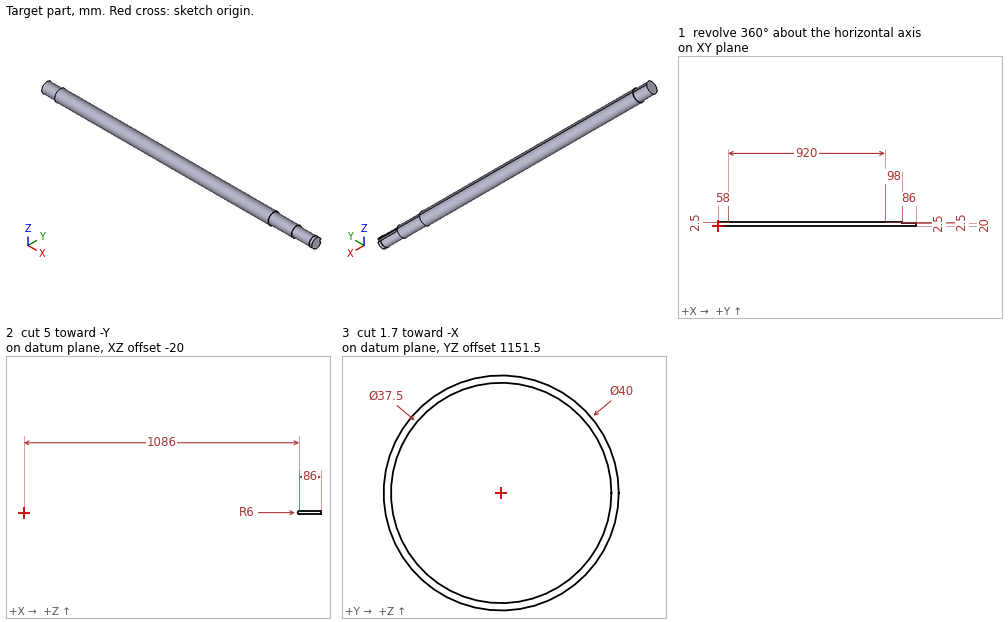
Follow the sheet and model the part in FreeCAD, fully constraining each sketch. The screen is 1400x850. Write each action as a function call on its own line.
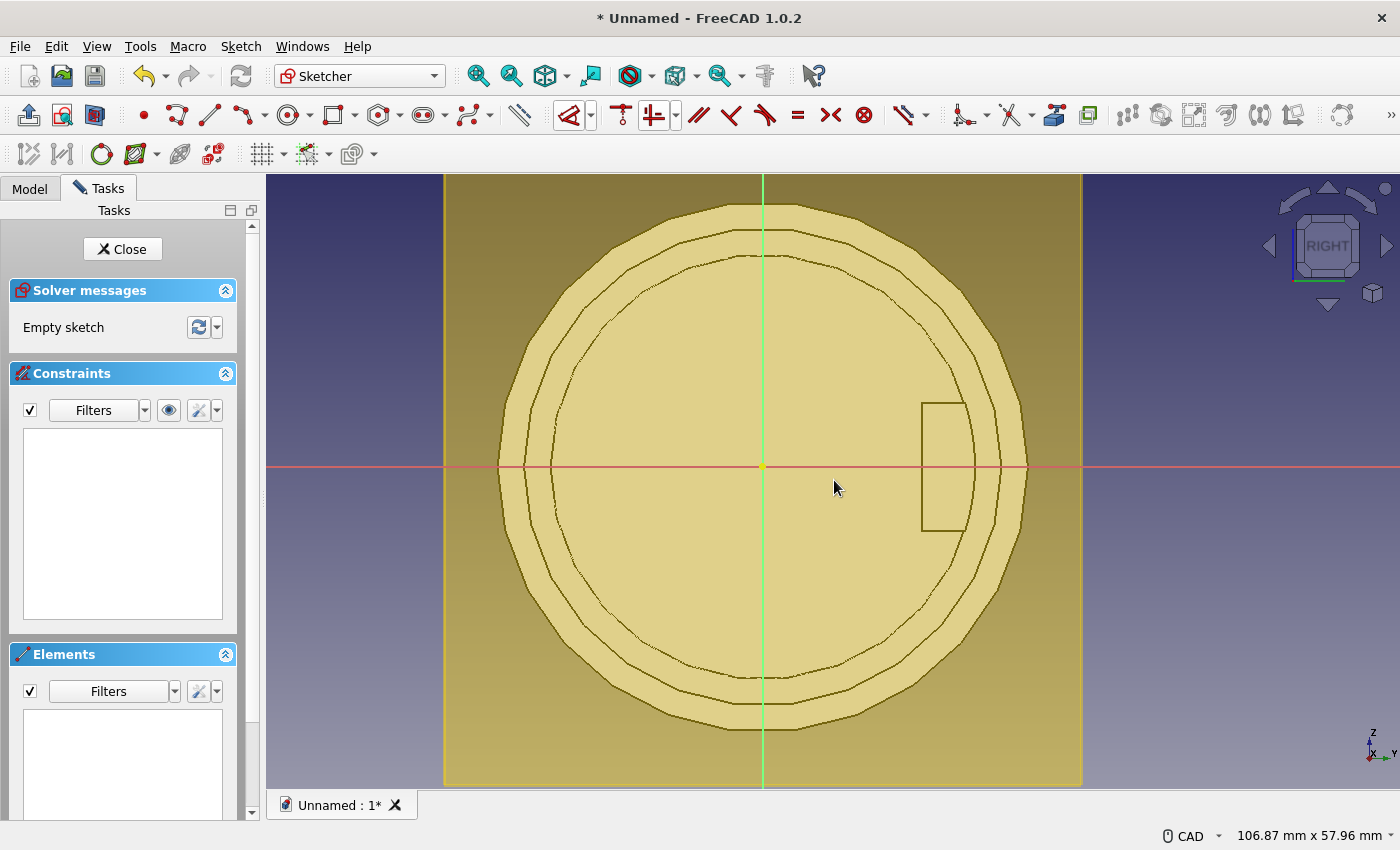
click(288, 116)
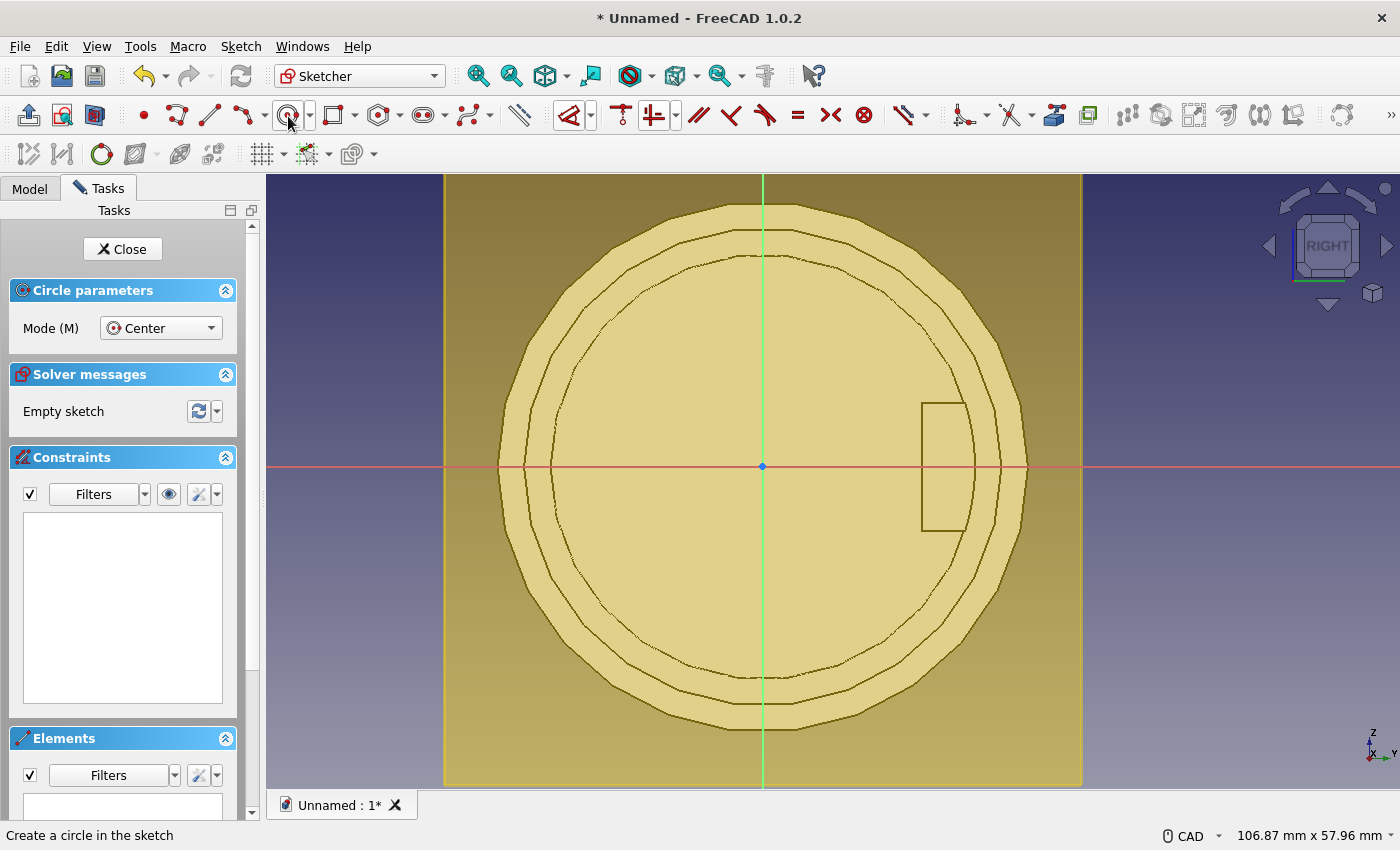
click(763, 467)
click(913, 317)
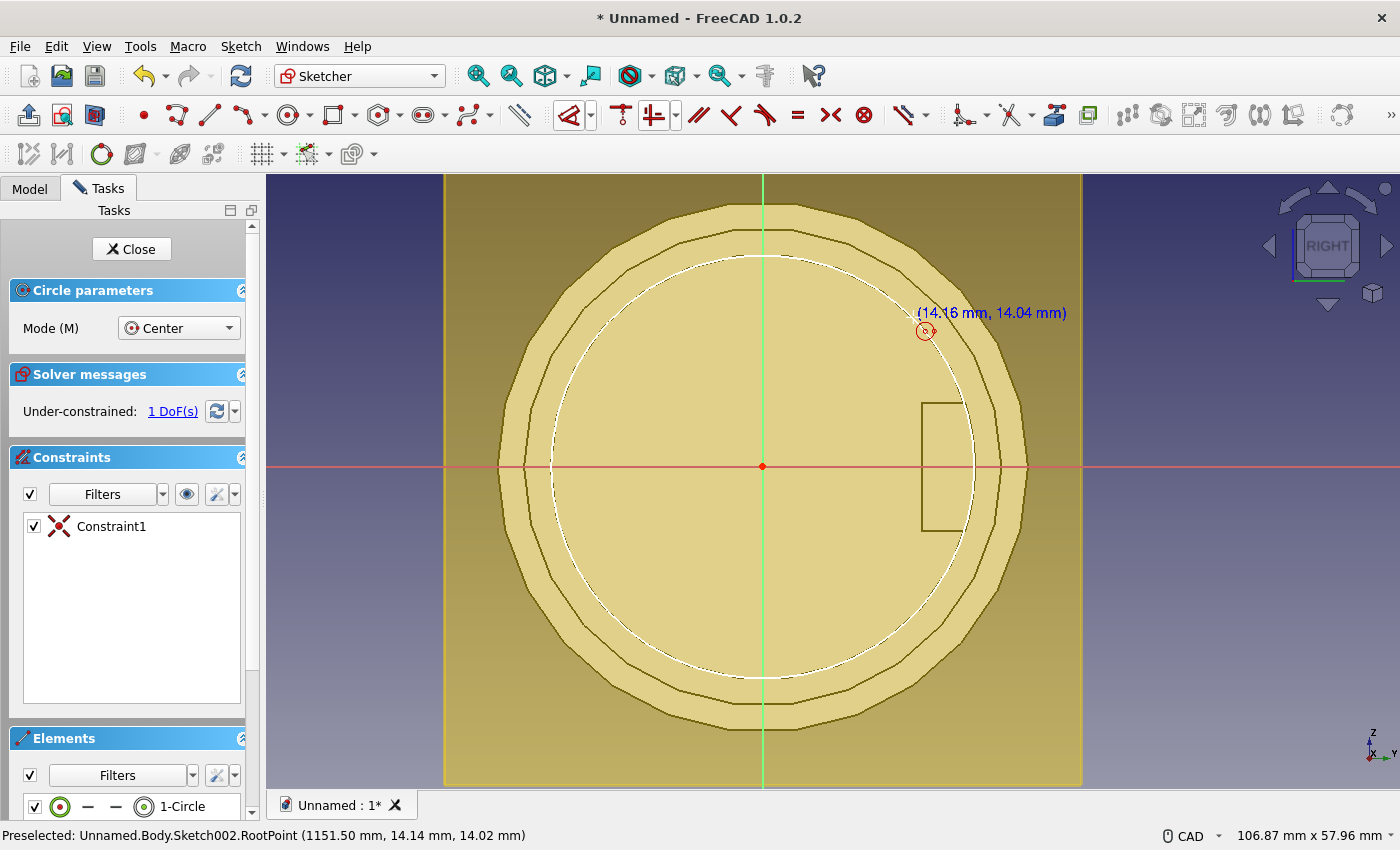
click(763, 467)
click(903, 326)
key(Escape)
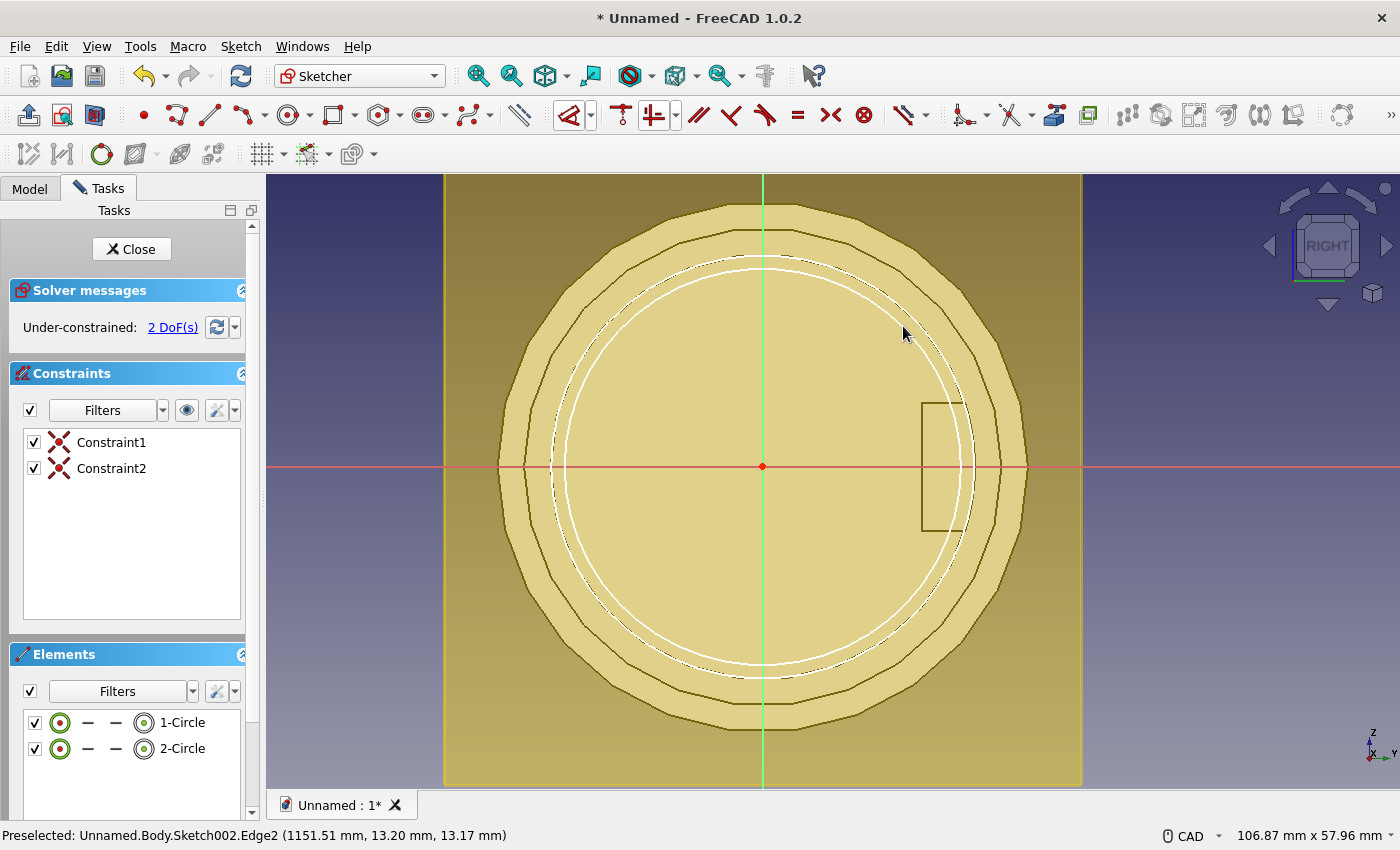
click(912, 317)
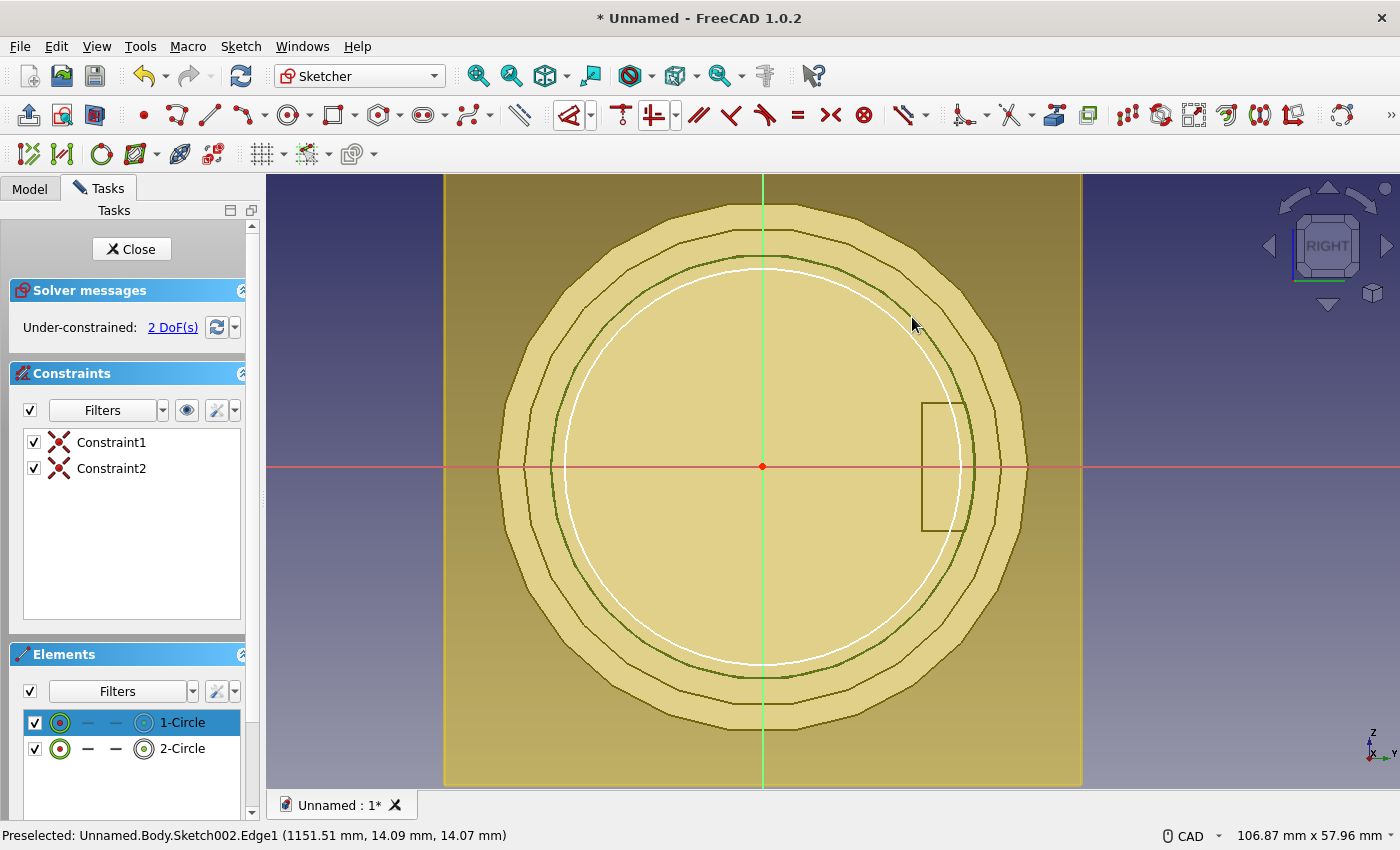
click(590, 116)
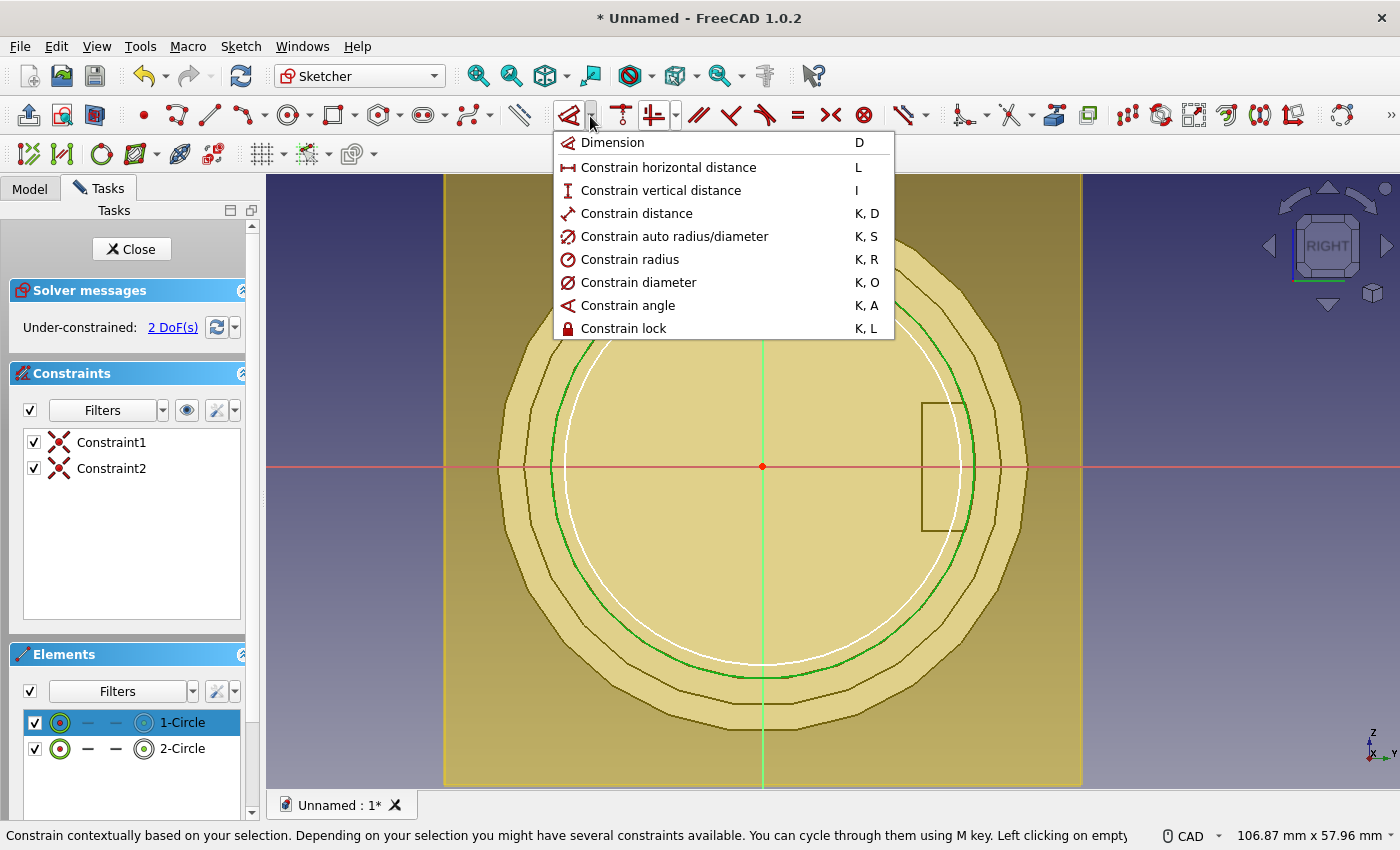
click(724, 282)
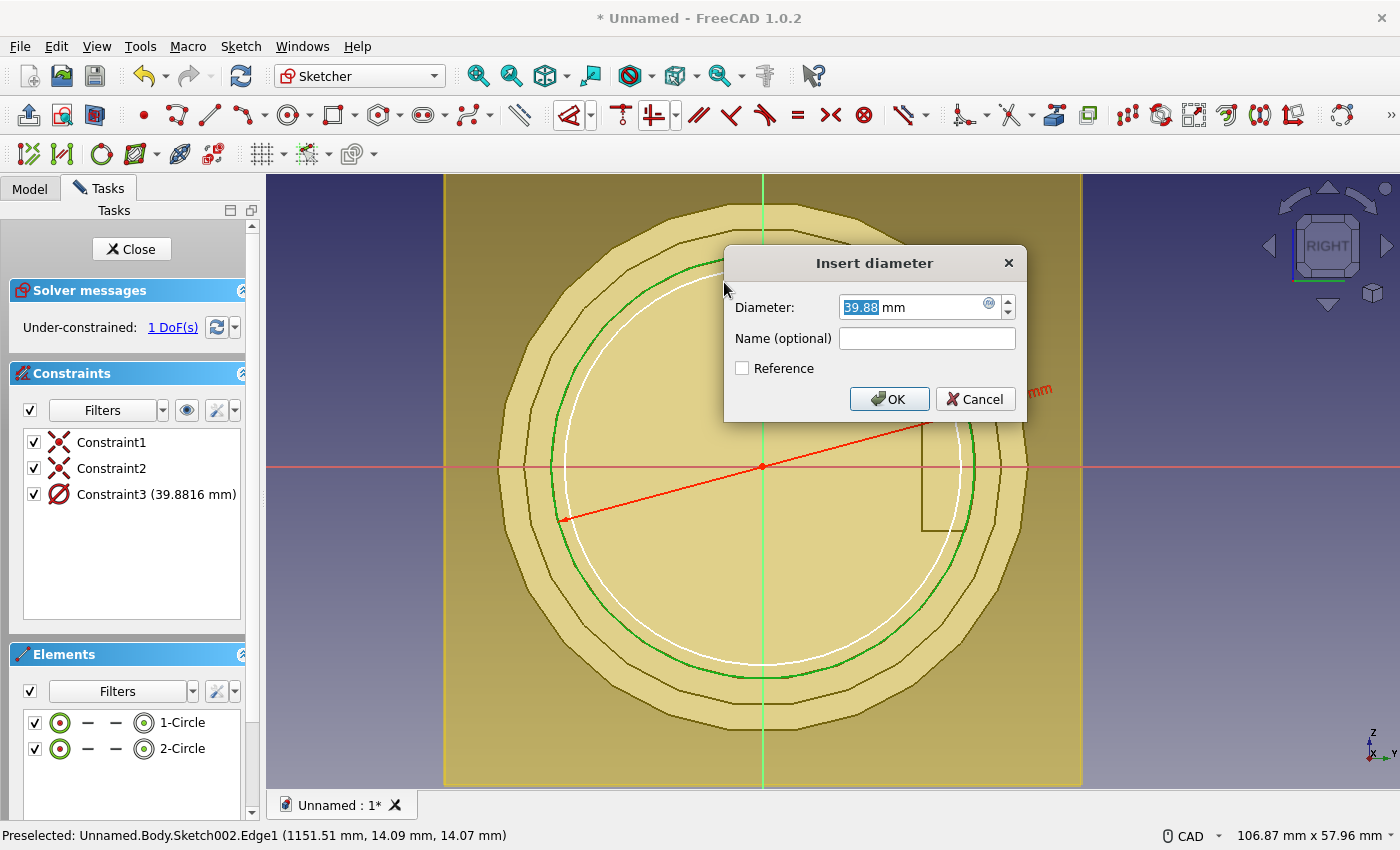
text(40)
key(Return)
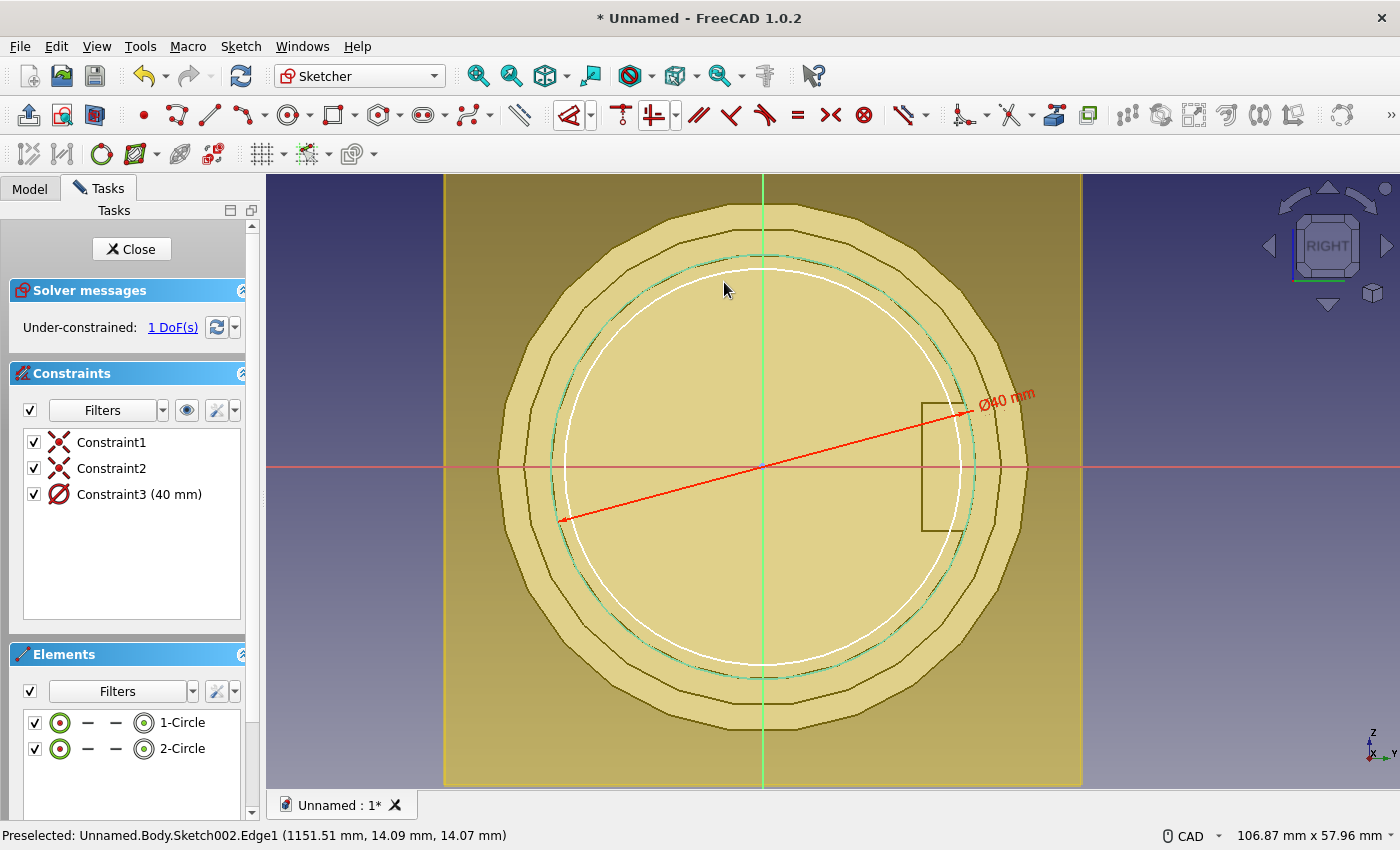
click(902, 326)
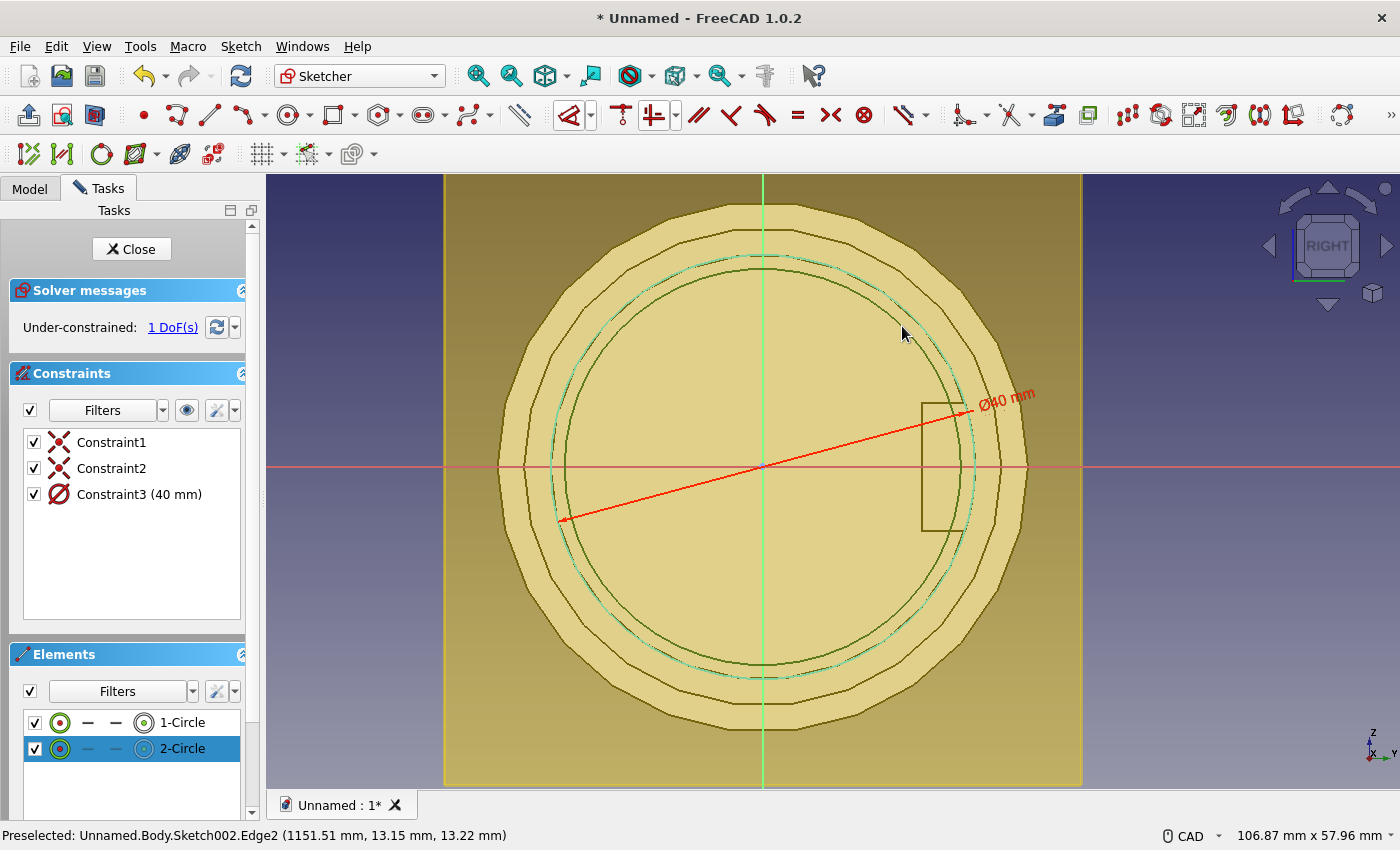
click(590, 116)